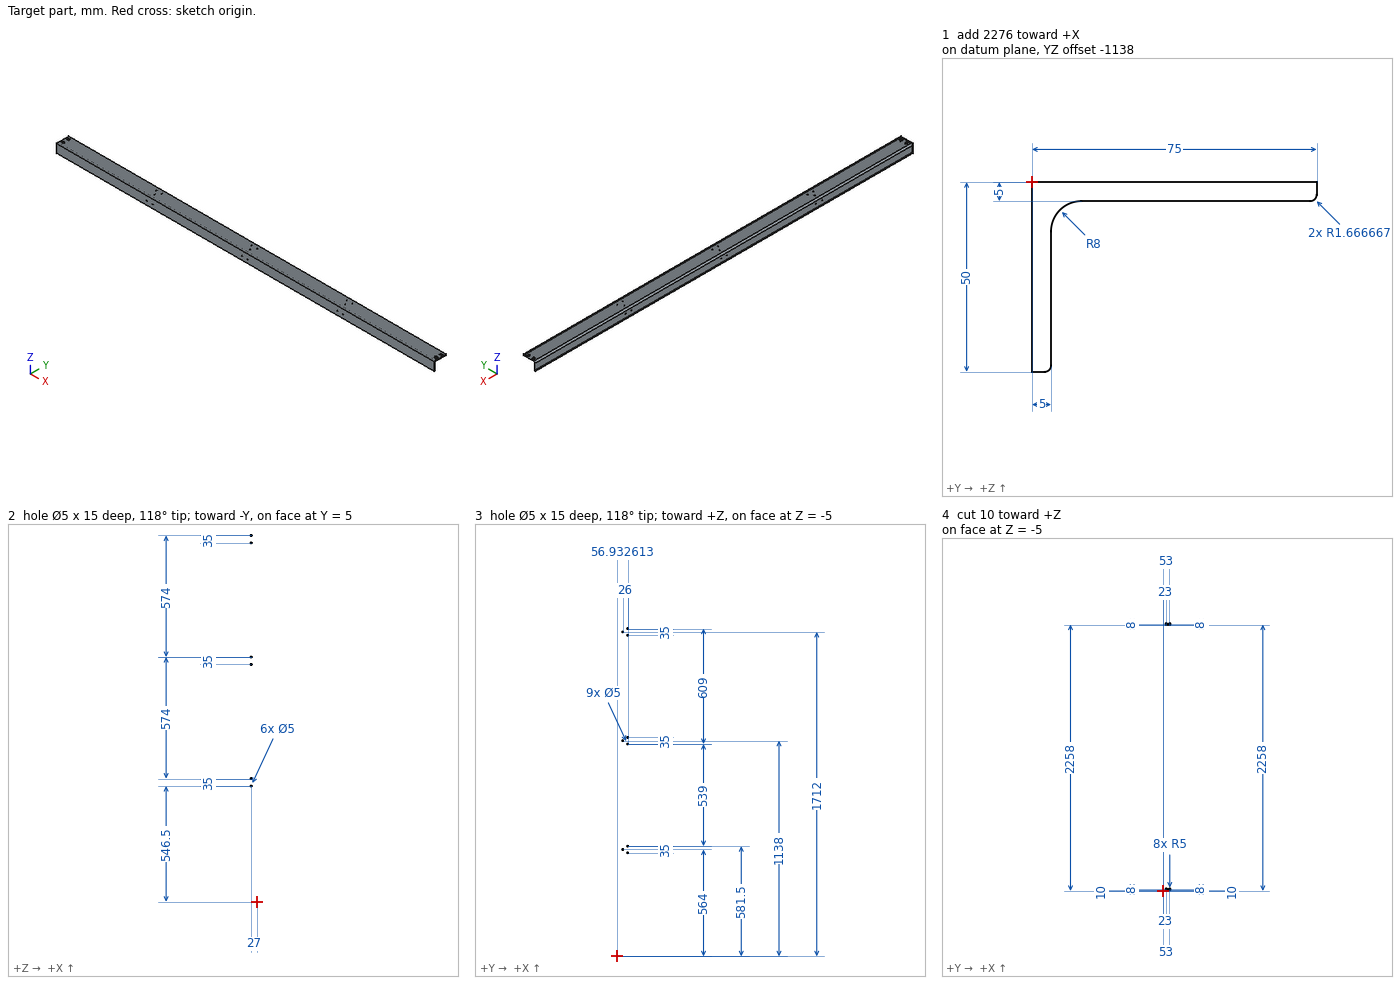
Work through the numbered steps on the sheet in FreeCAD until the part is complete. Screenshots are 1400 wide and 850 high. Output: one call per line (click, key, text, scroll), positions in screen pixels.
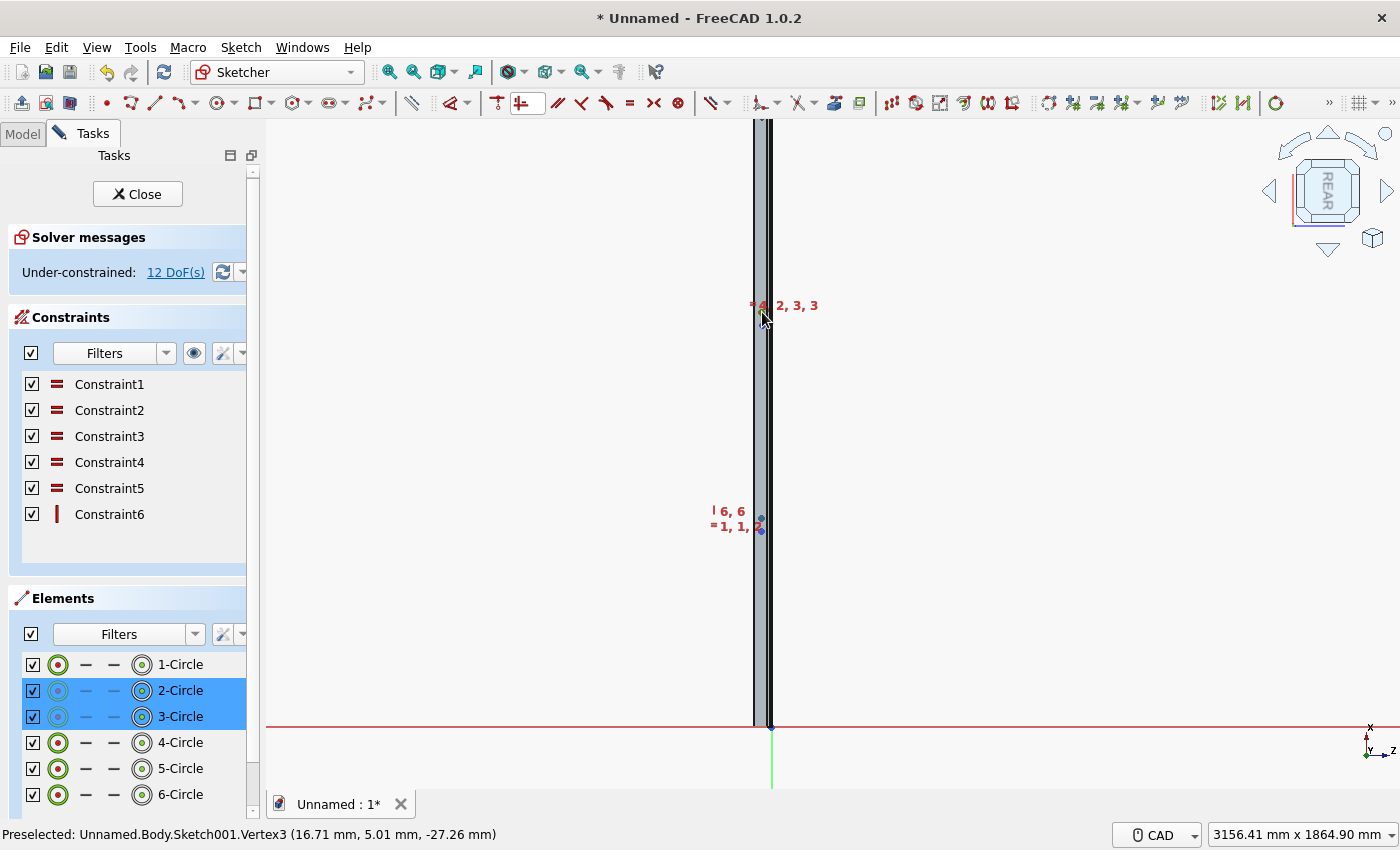
click(540, 104)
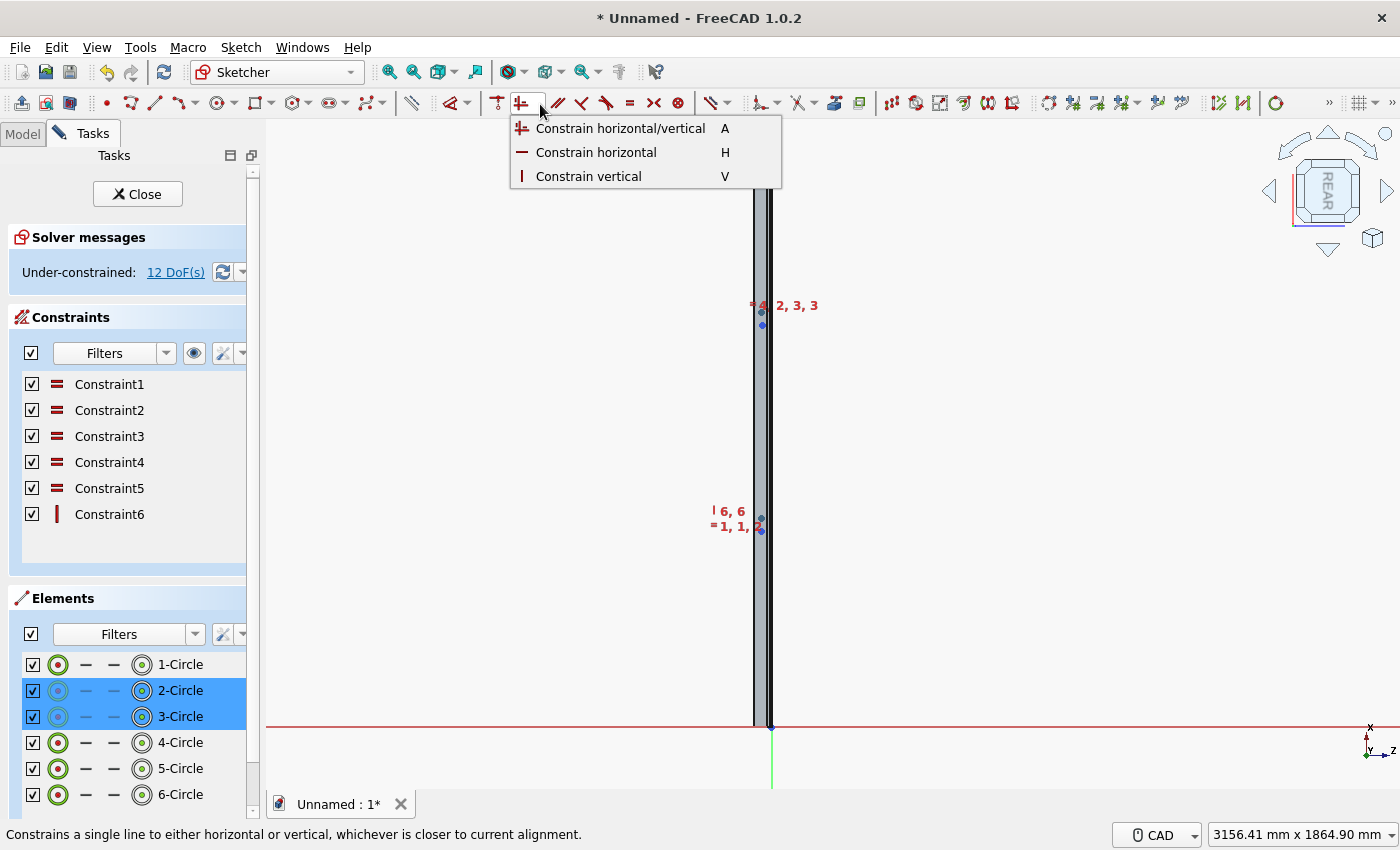
click(646, 176)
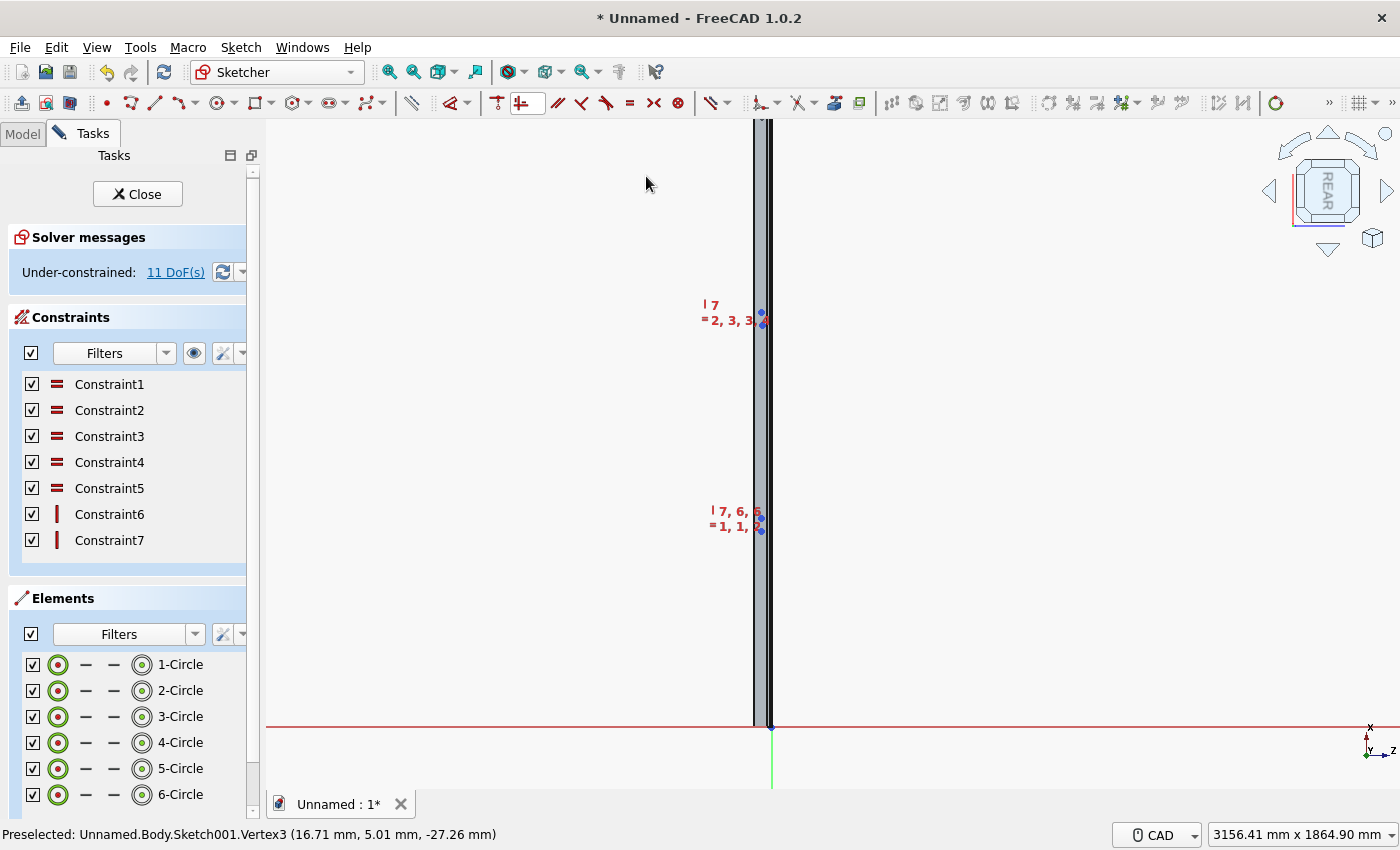
scroll(762, 312, up, 4)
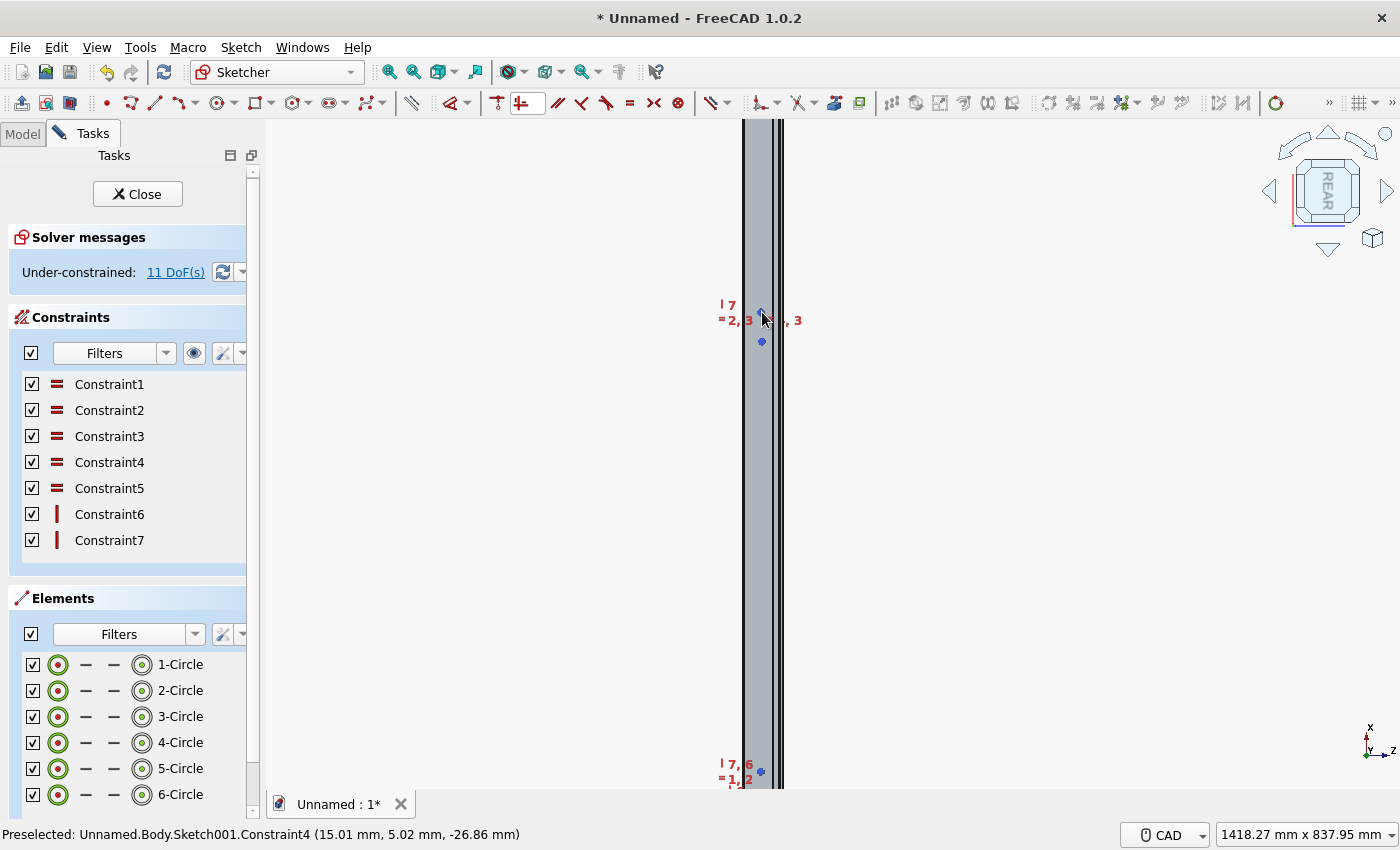
click(761, 313)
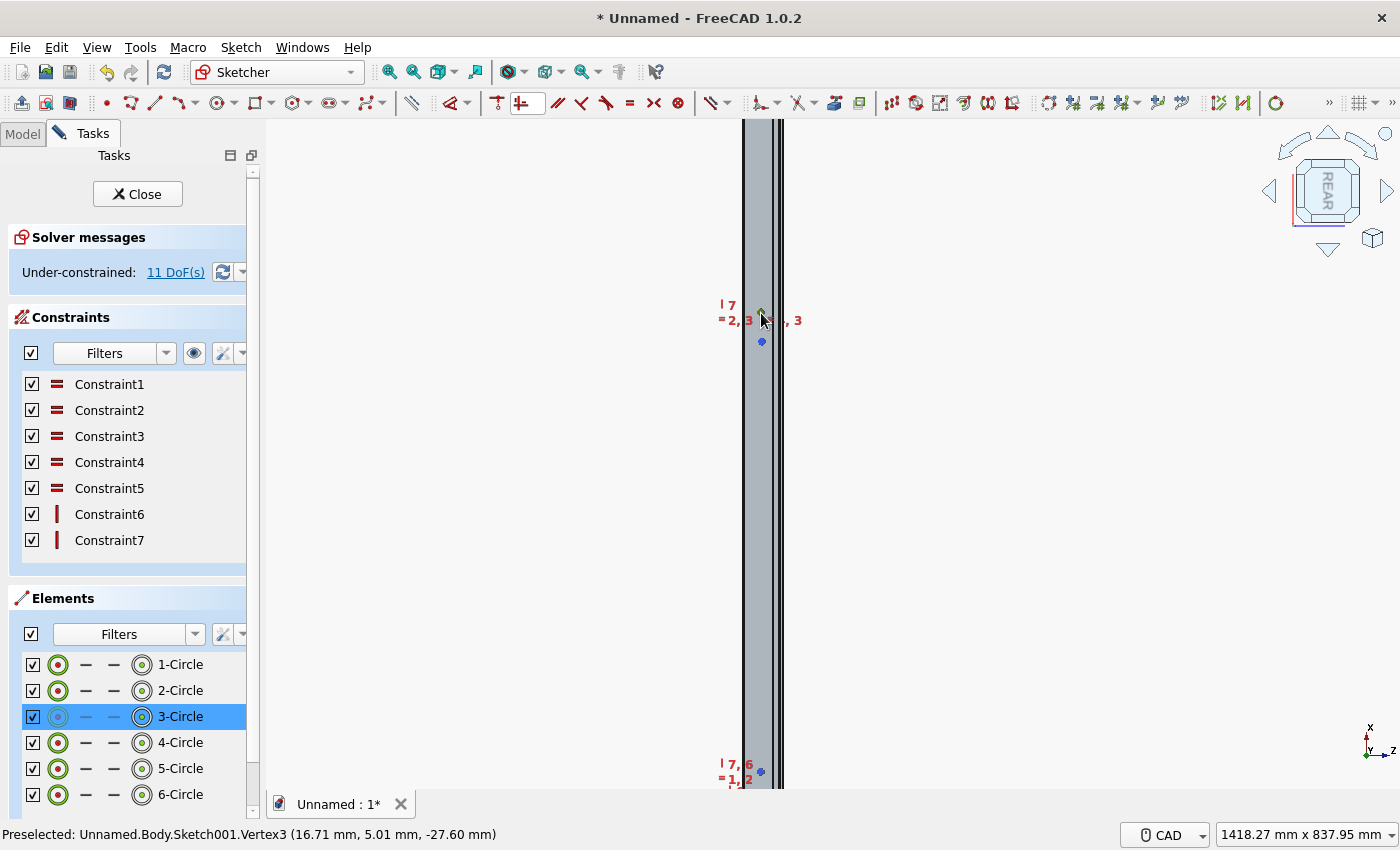
click(762, 342)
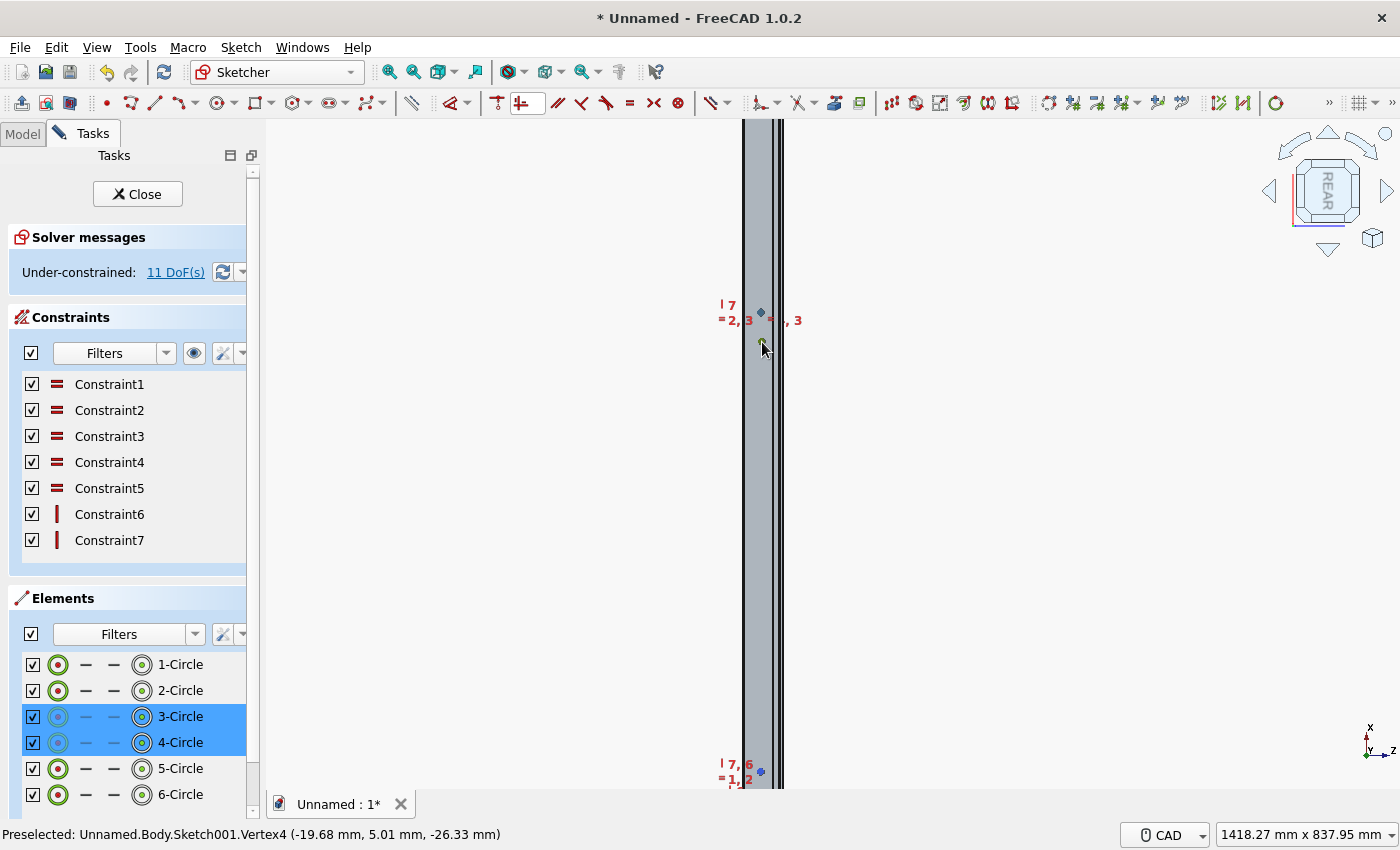
click(540, 104)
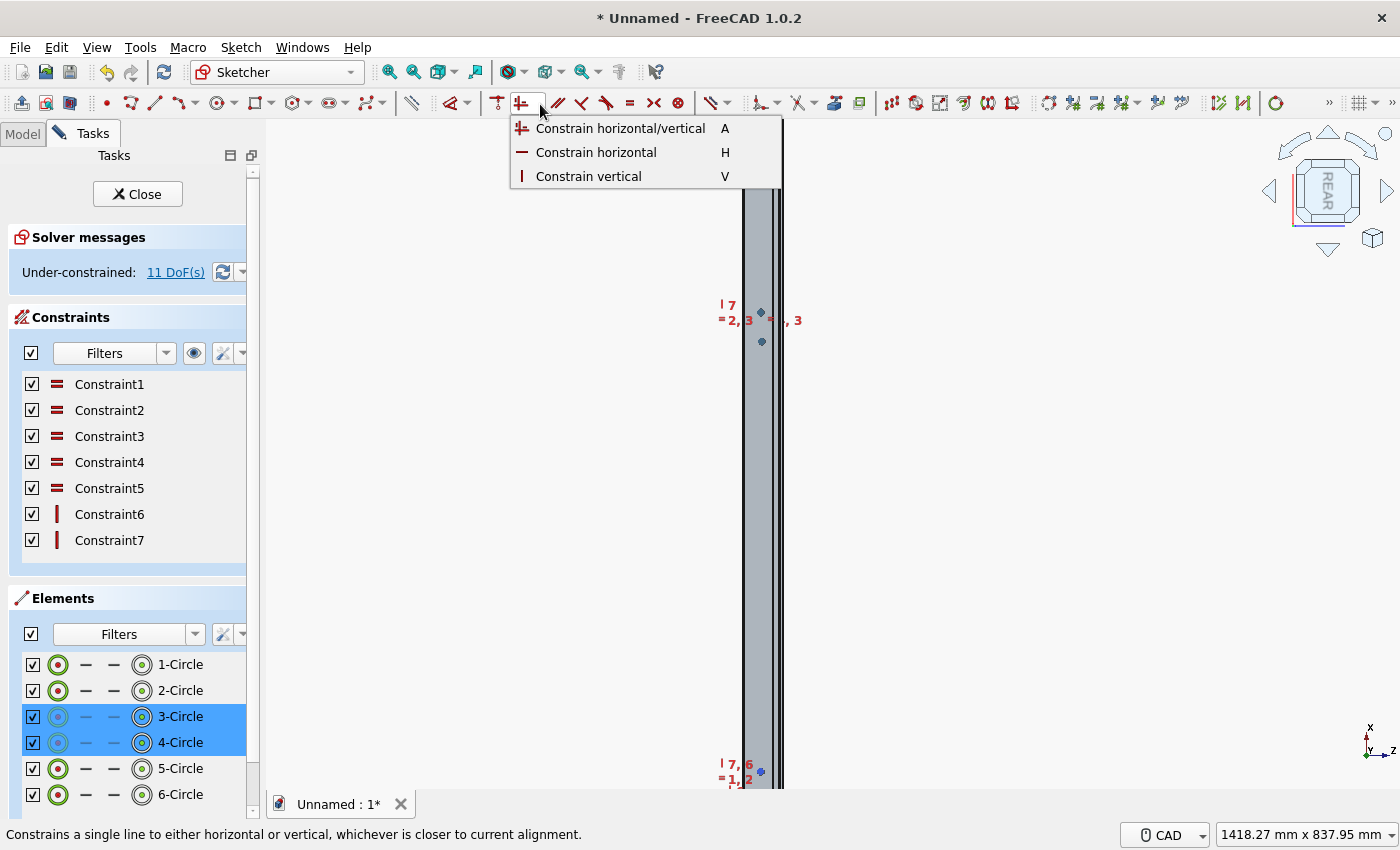
click(646, 176)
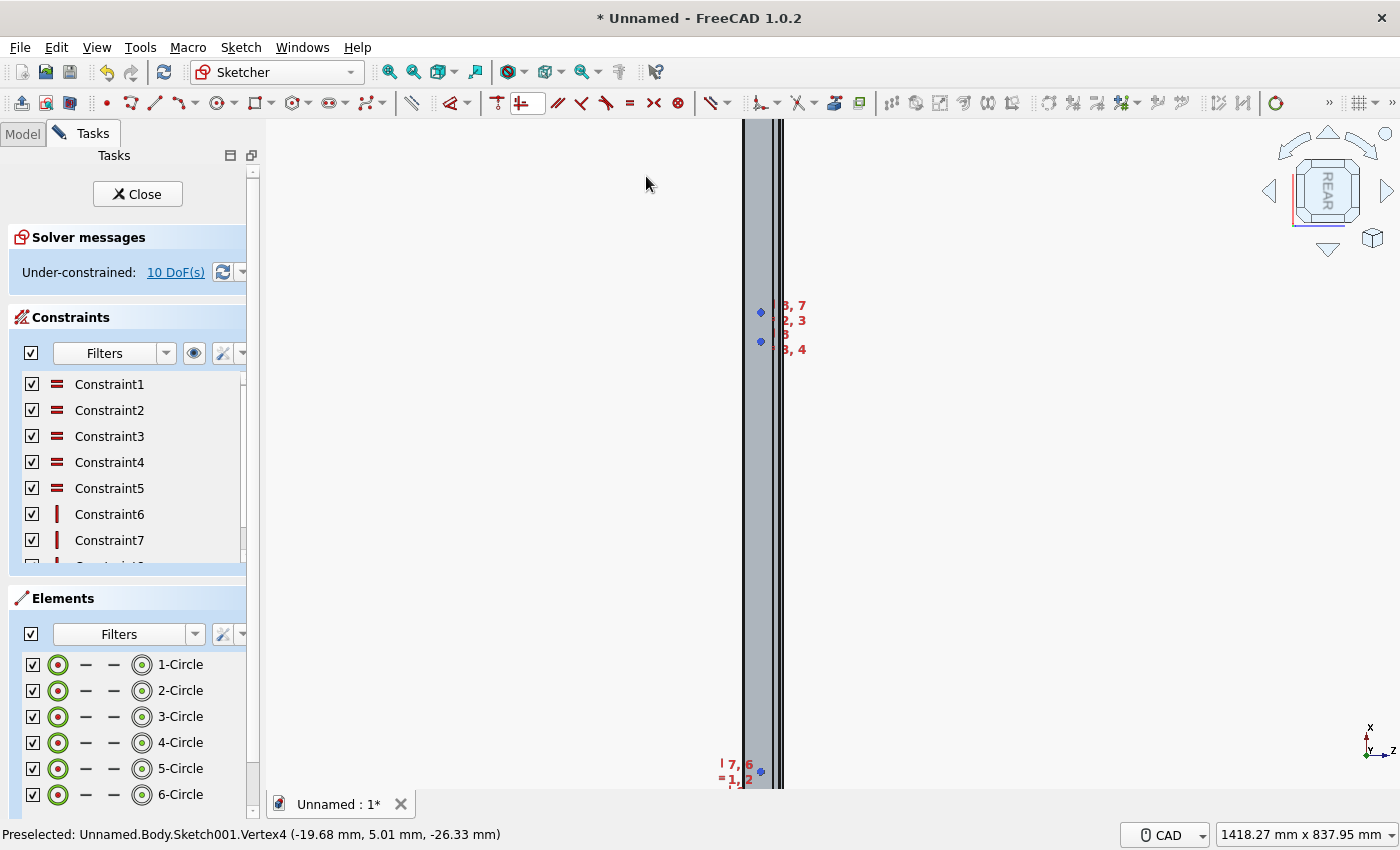
click(761, 313)